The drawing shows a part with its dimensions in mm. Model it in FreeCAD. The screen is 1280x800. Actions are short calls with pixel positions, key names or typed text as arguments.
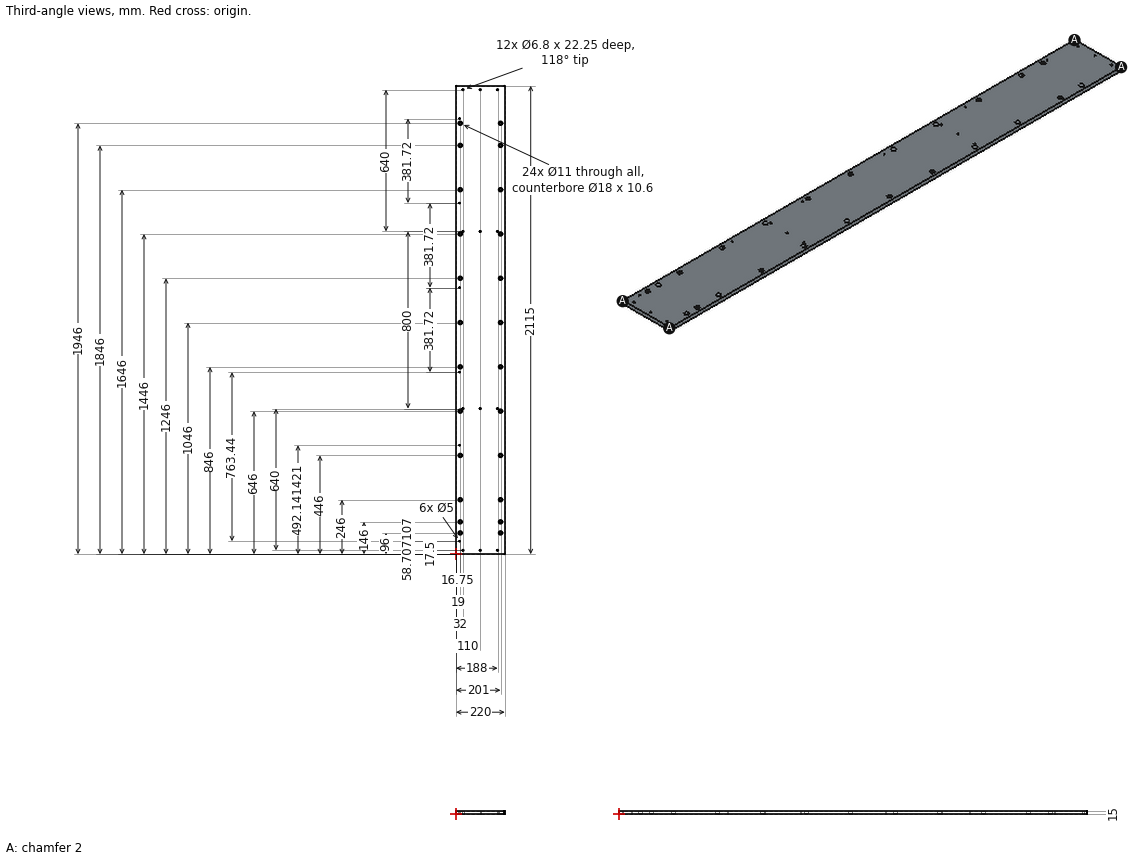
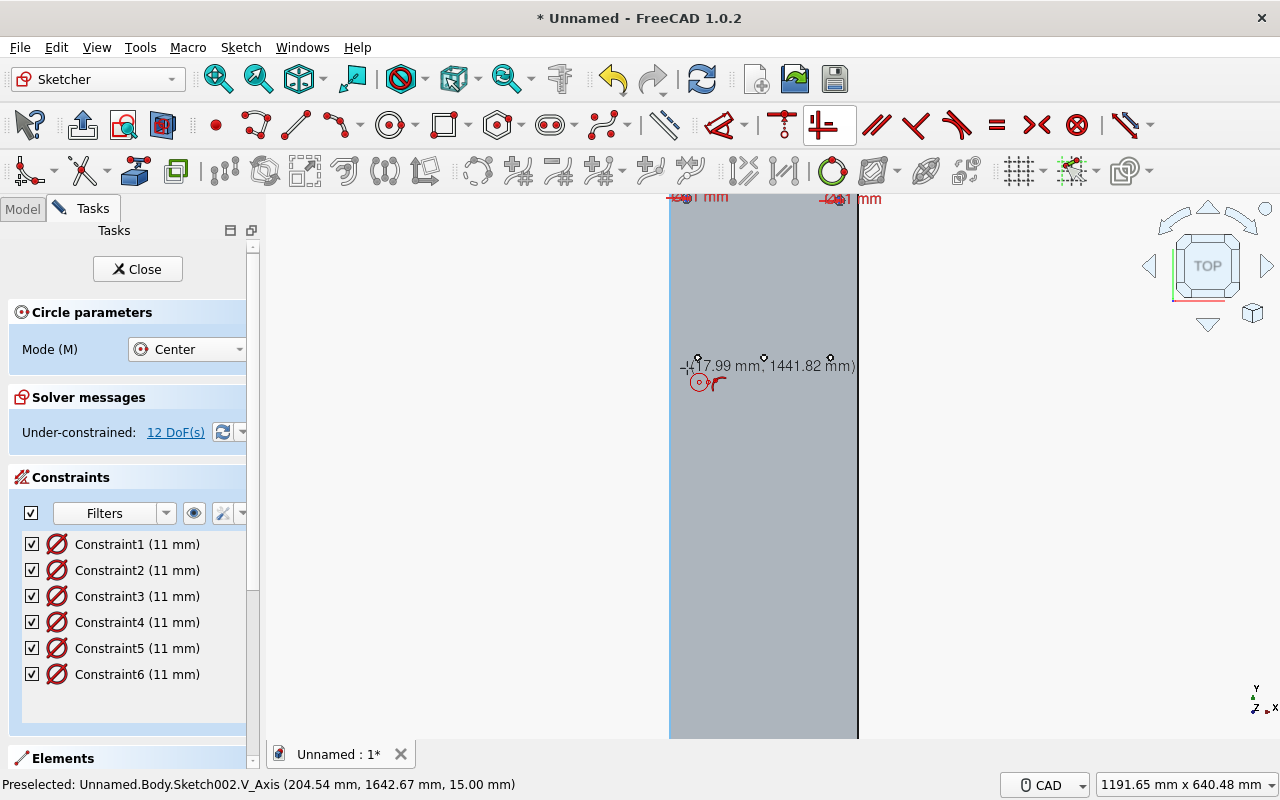
click(687, 368)
move(690, 364)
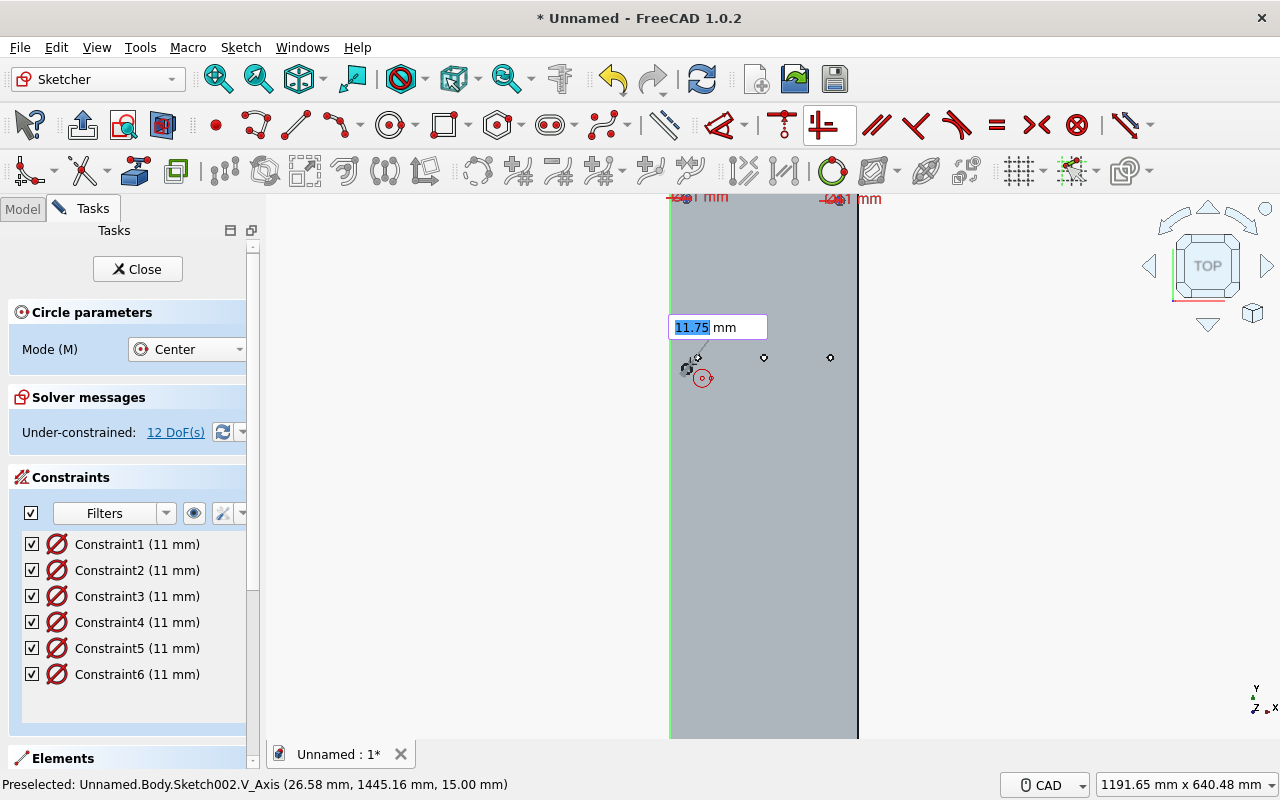
text(11)
key(Return)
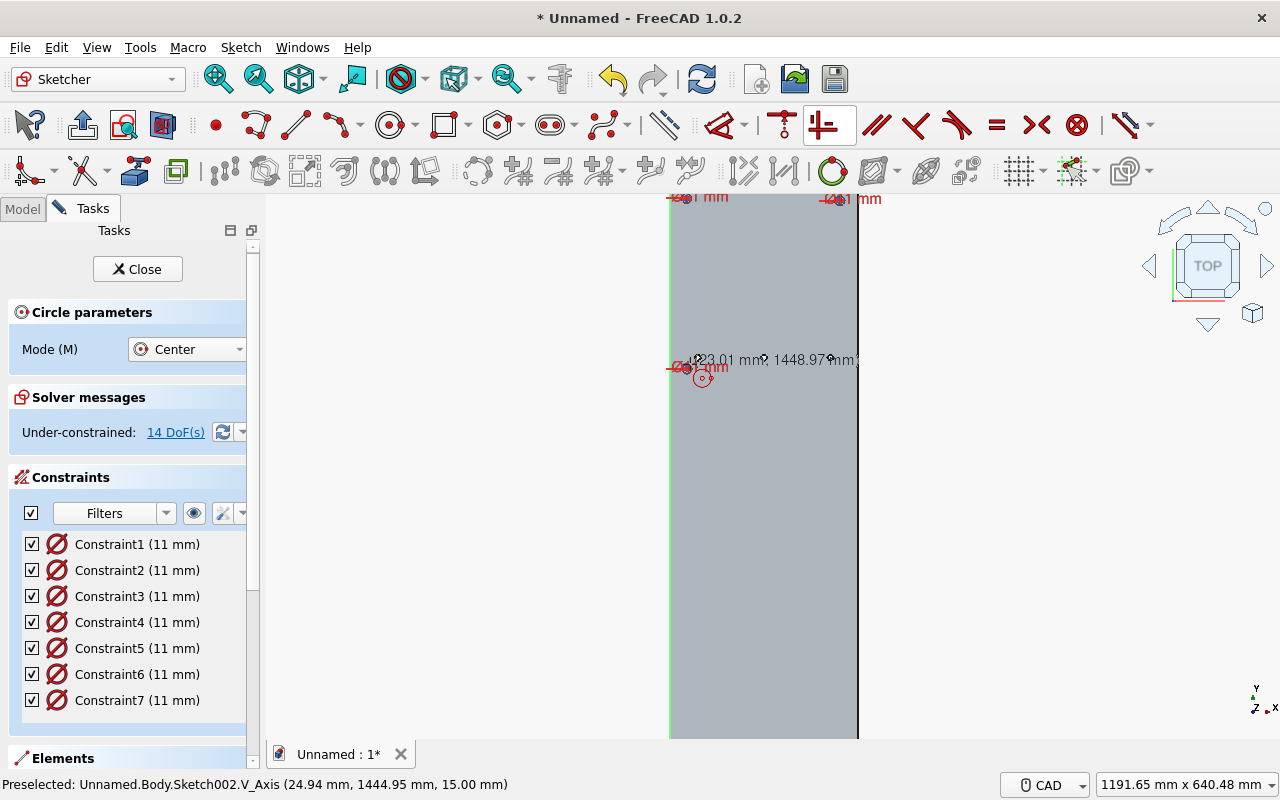
scroll(841, 368, up, 8)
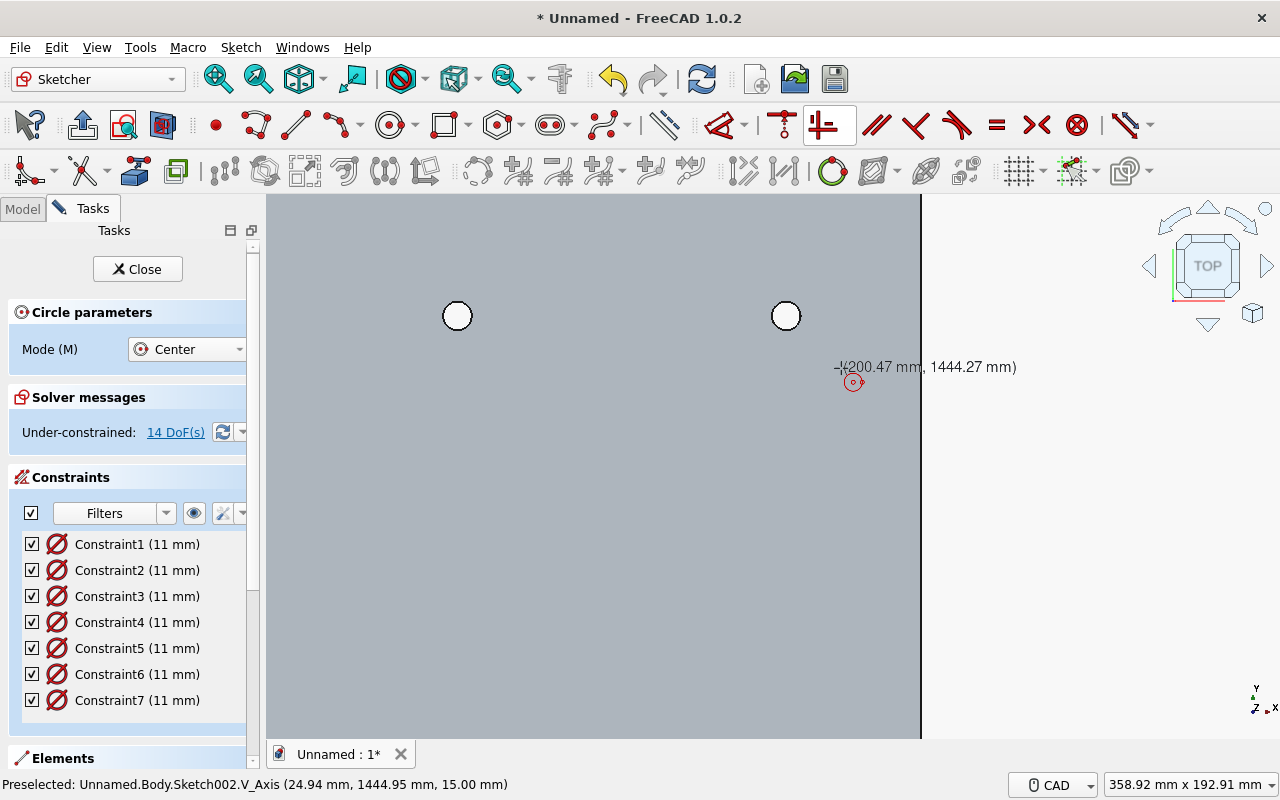
scroll(719, 368, down, 15)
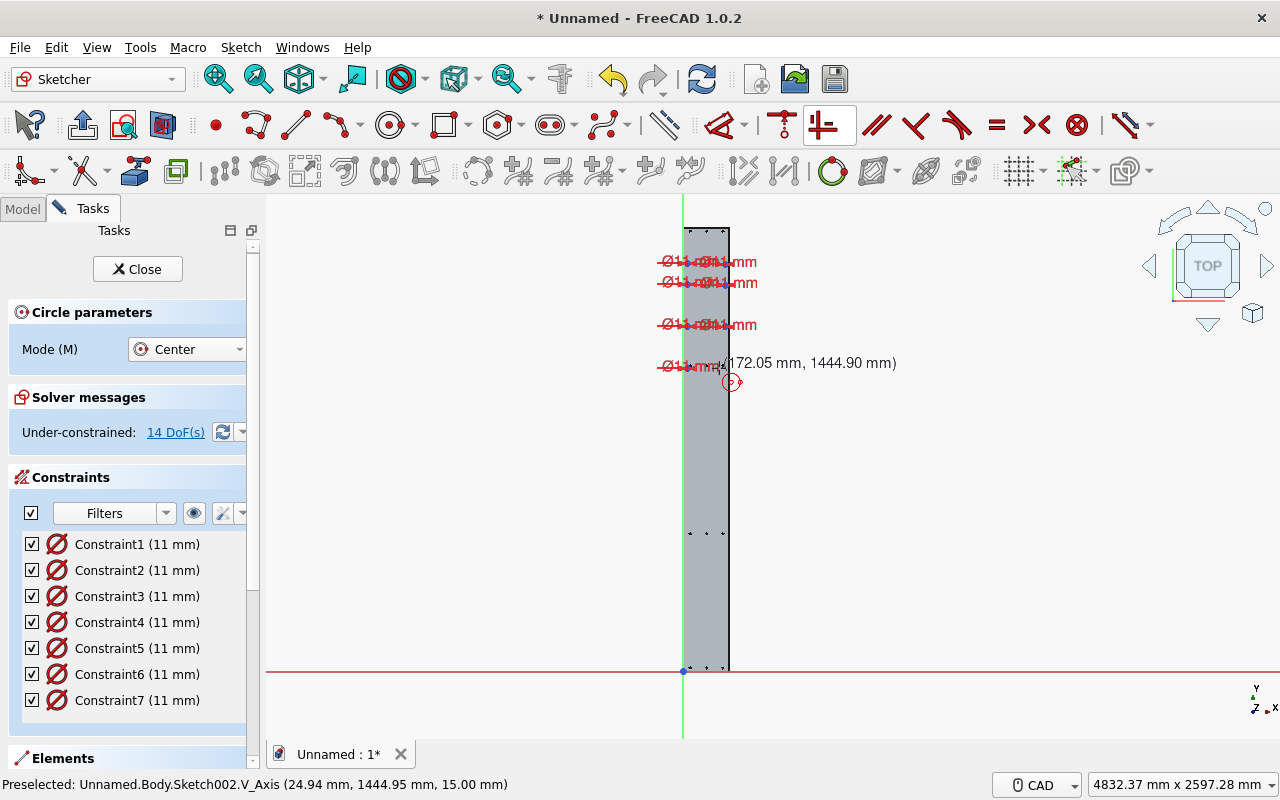
click(725, 368)
move(726, 367)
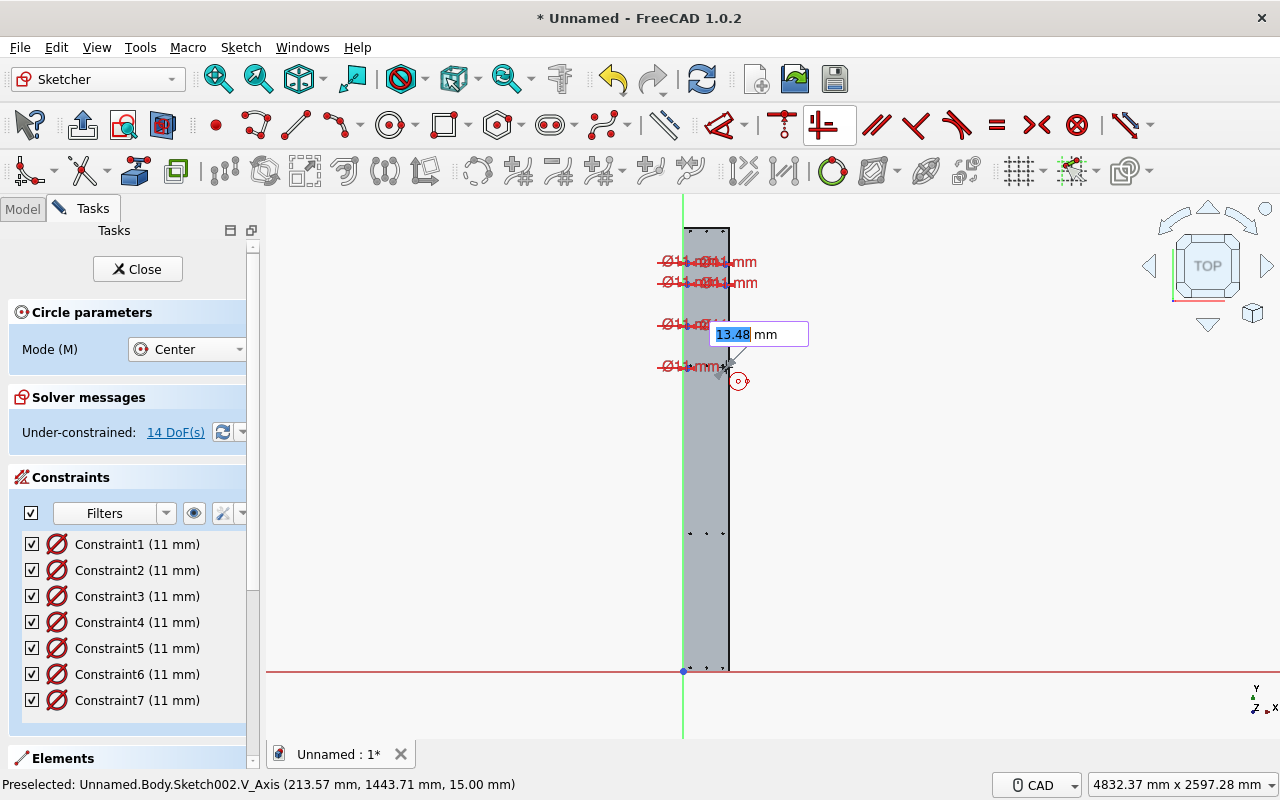
text(11)
key(Return)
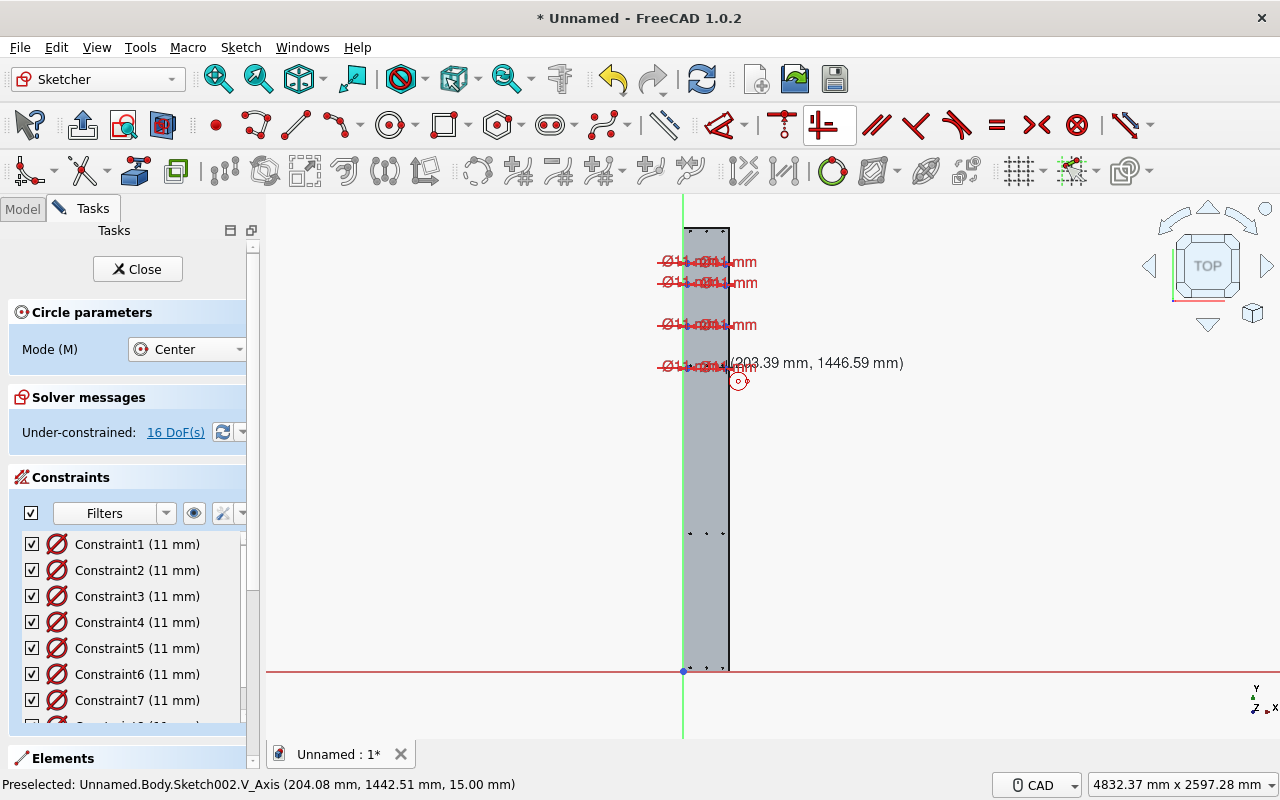
scroll(687, 410, up, 15)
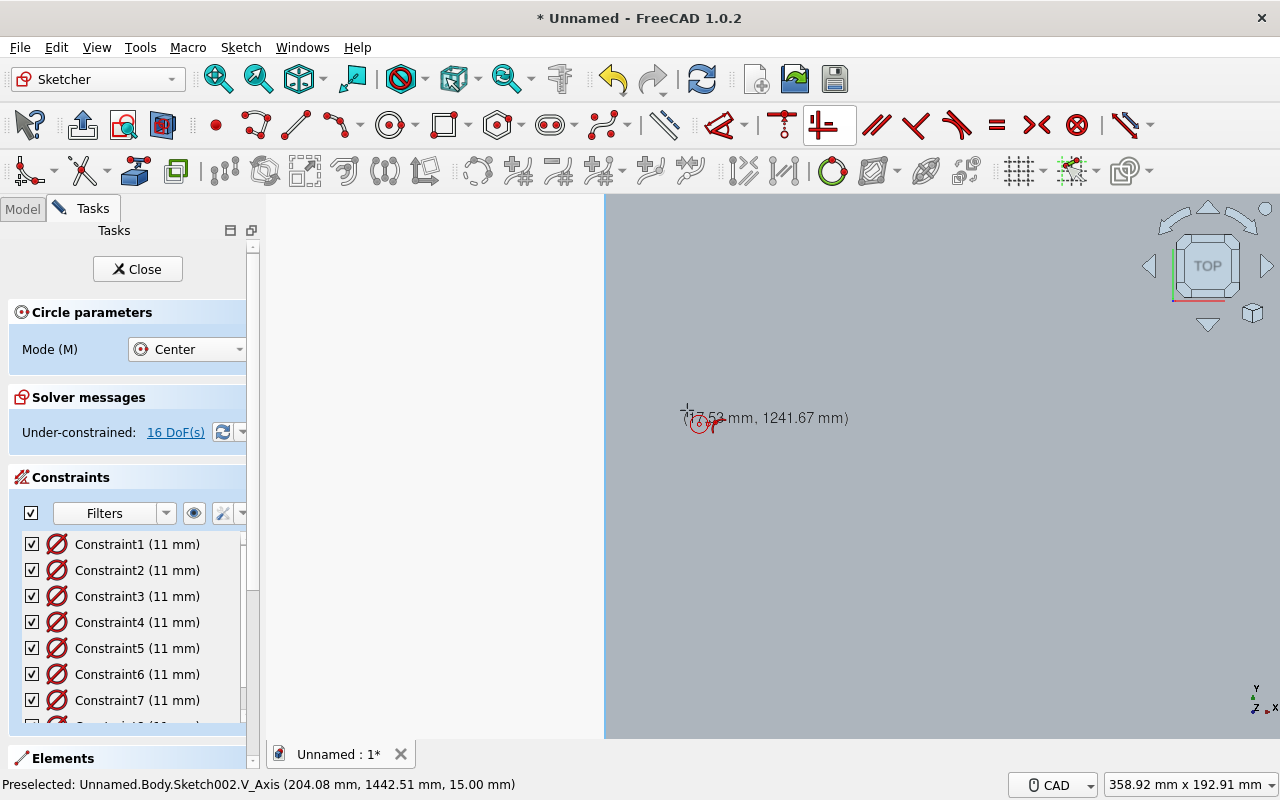
scroll(687, 410, down, 15)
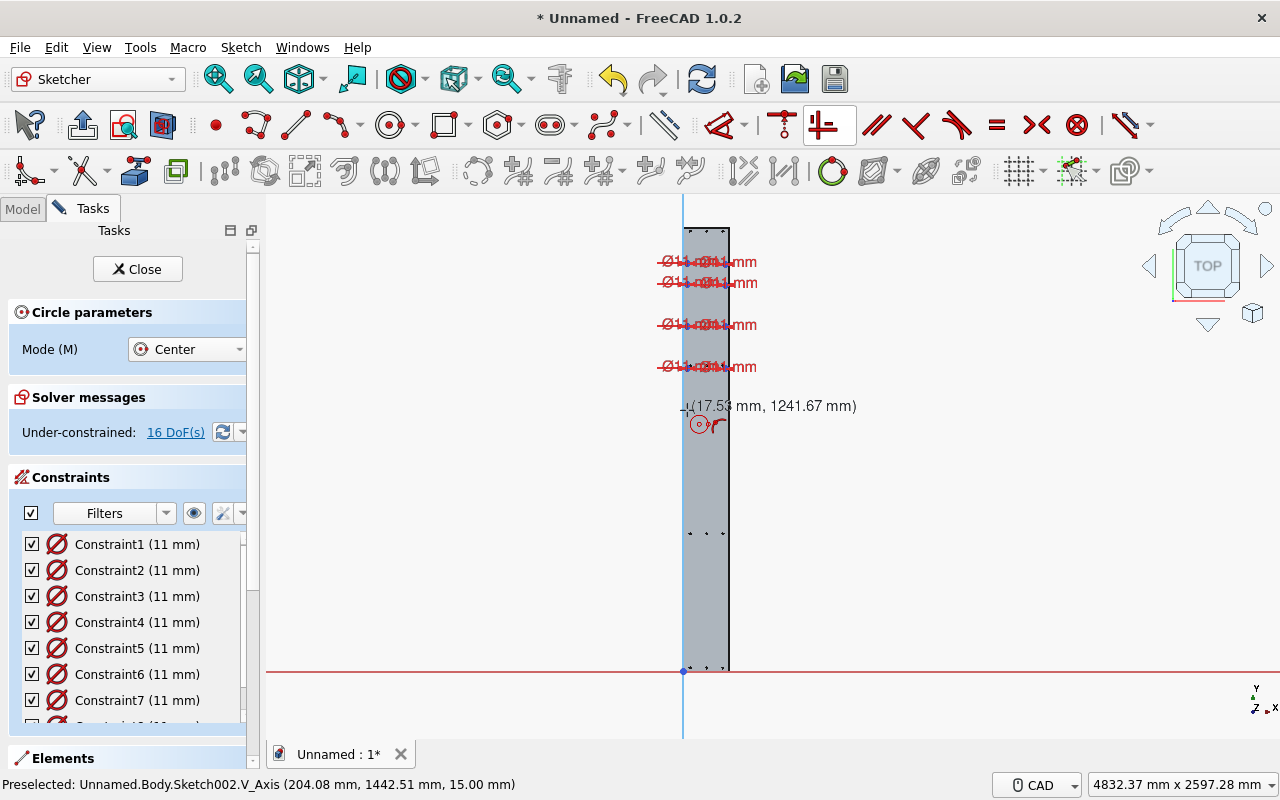
scroll(687, 410, up, 7)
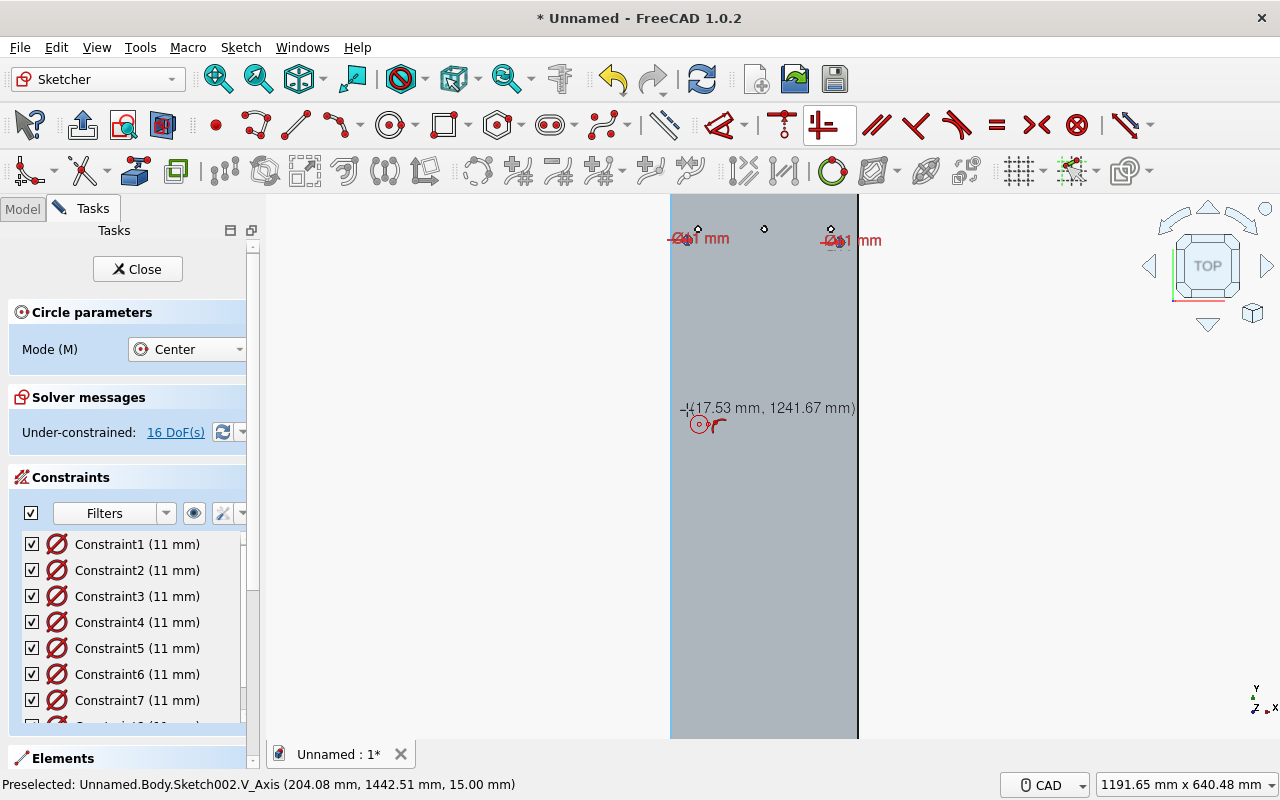
click(687, 409)
move(690, 406)